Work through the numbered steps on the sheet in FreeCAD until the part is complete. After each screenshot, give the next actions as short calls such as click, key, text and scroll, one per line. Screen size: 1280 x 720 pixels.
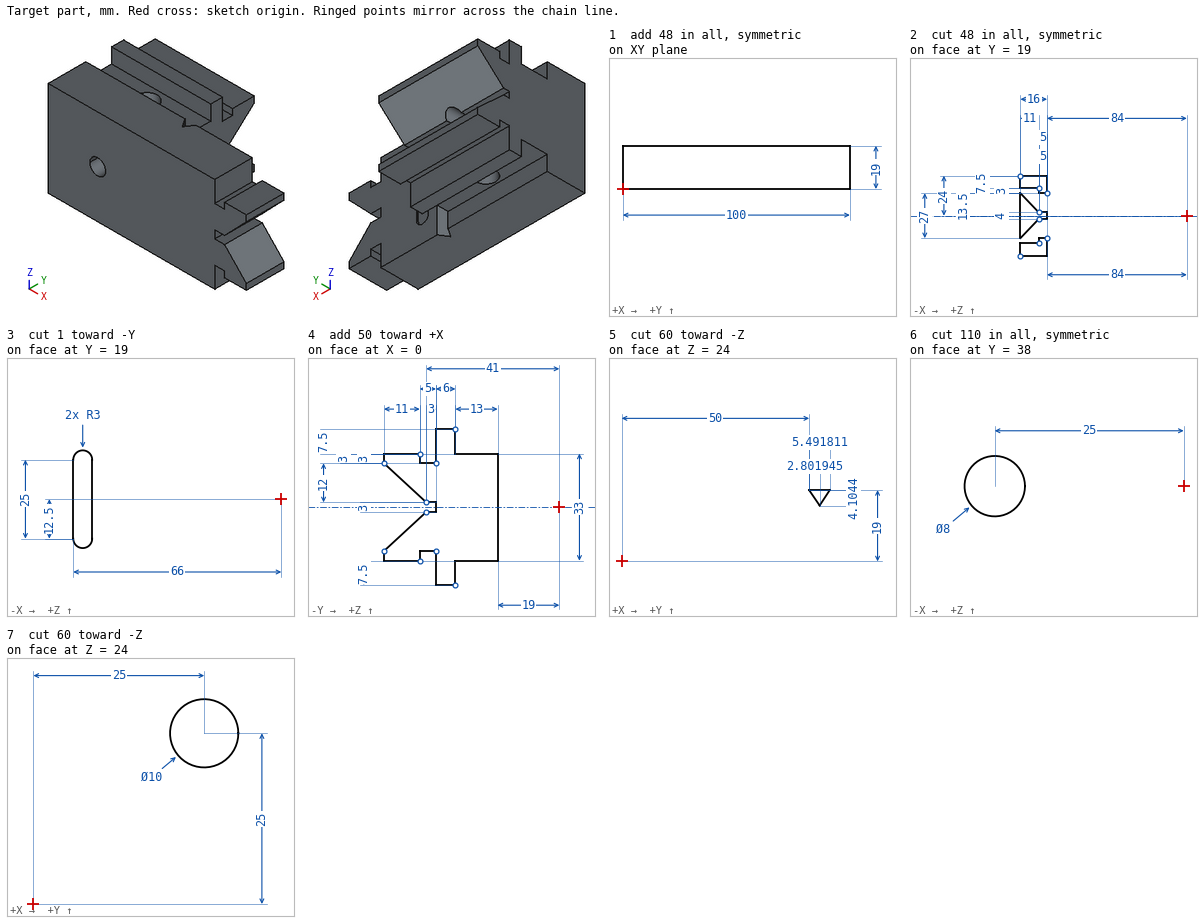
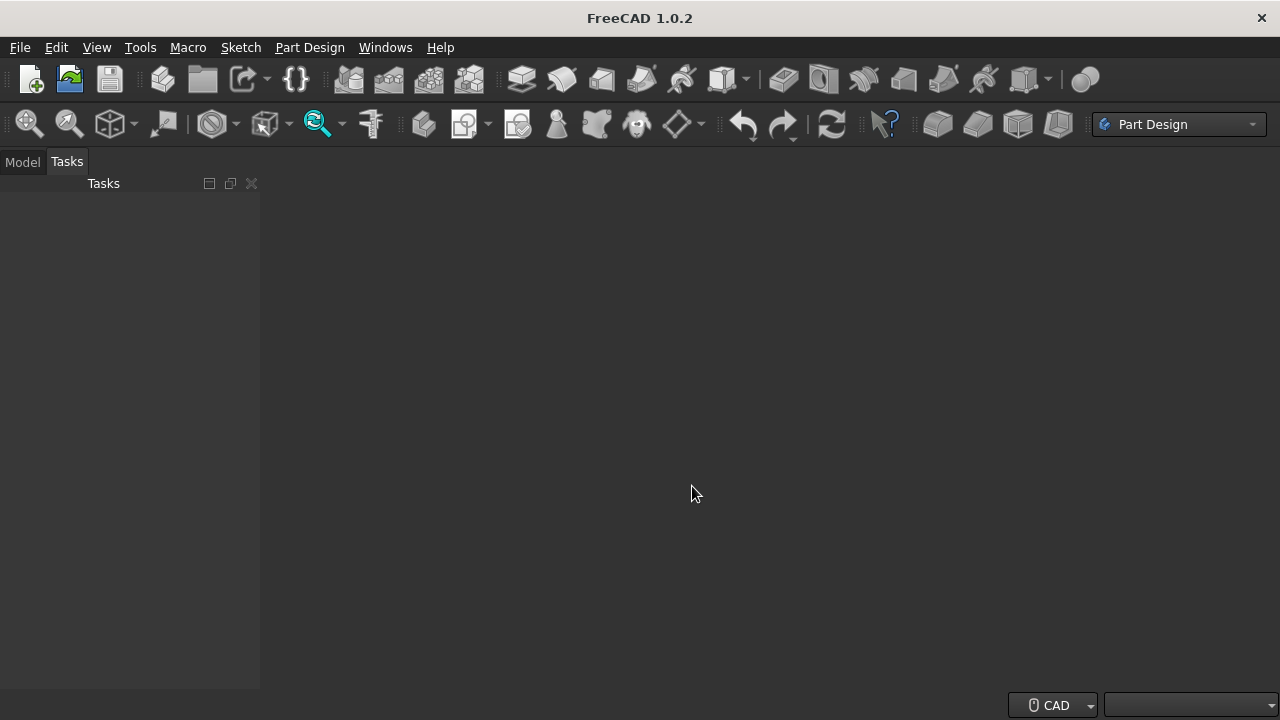
click(30, 80)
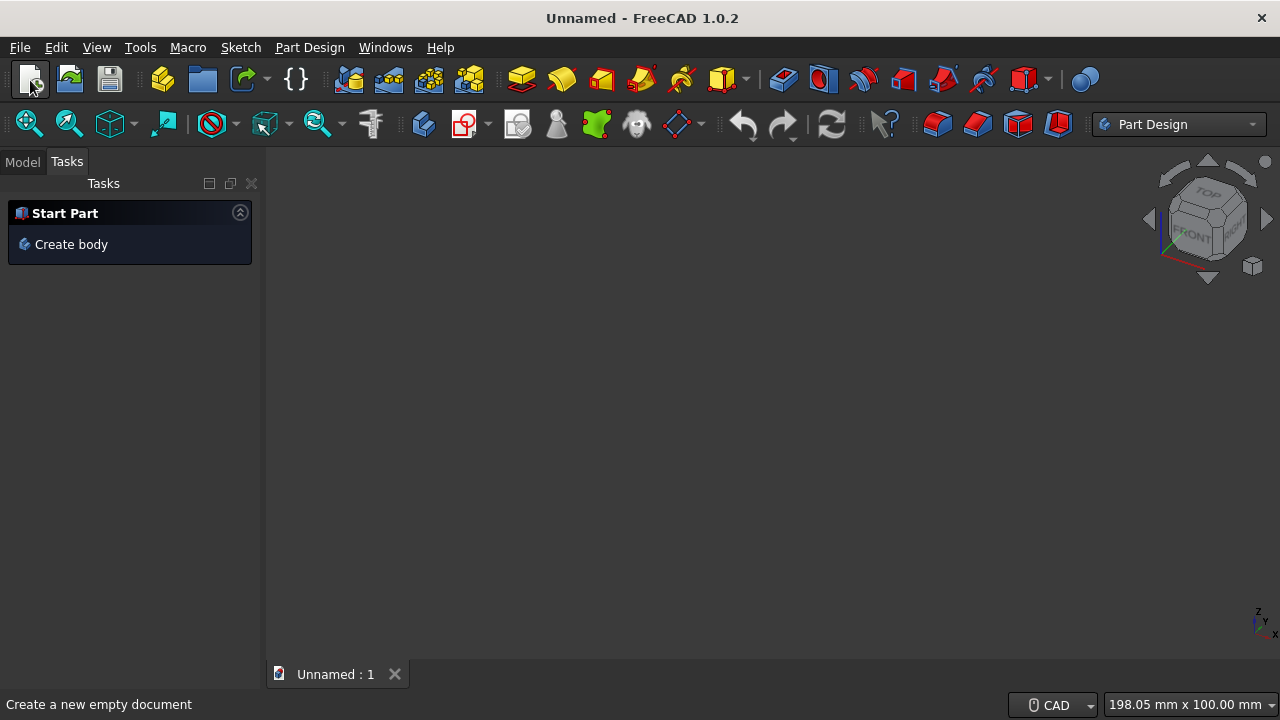
click(464, 124)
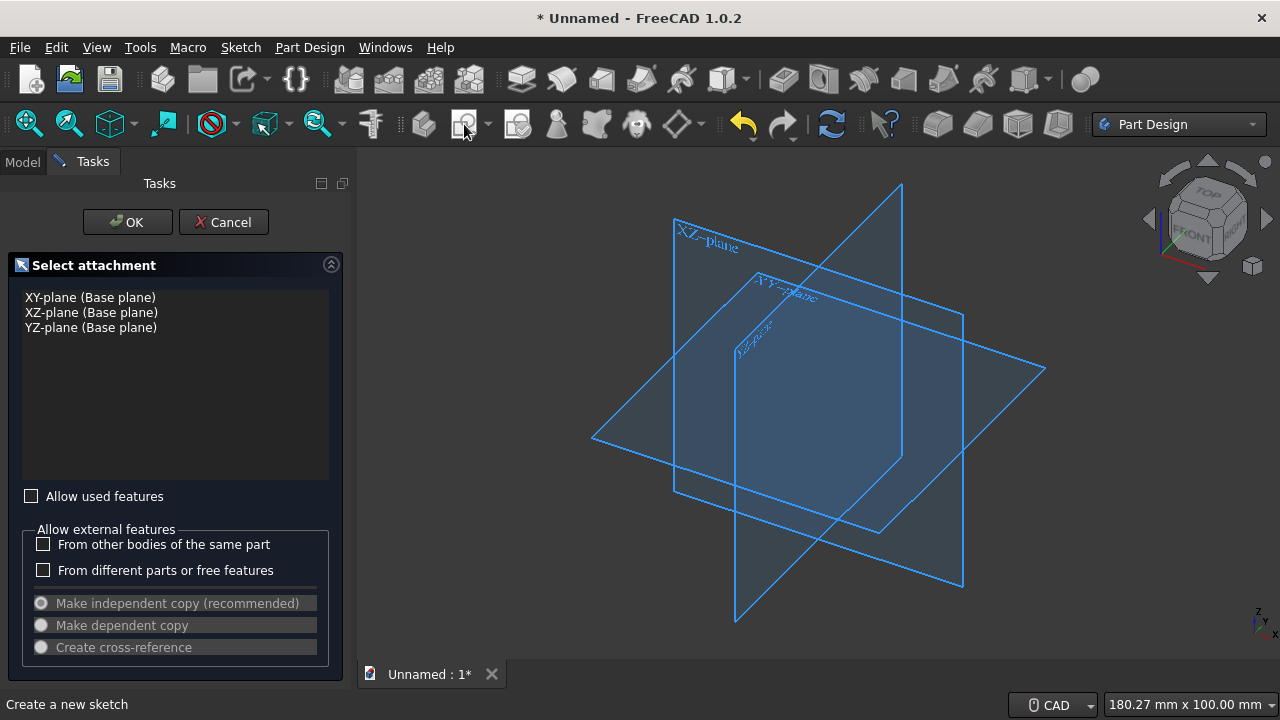
click(82, 298)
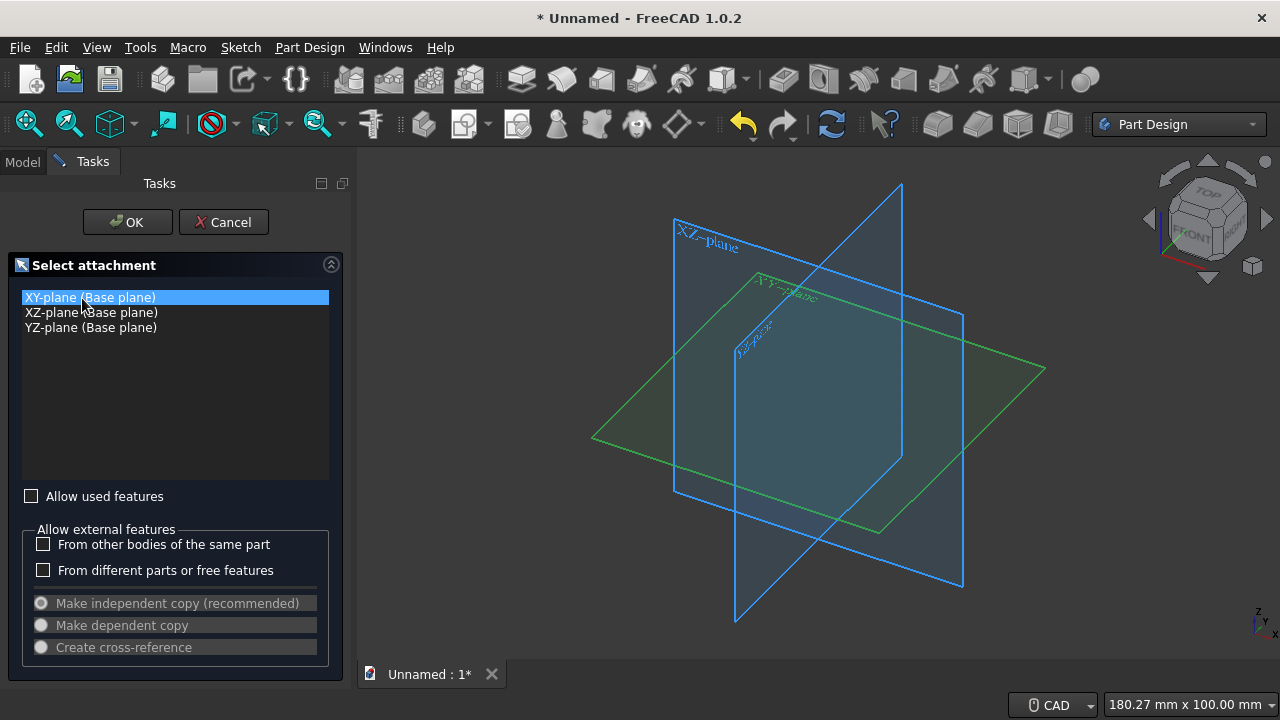
click(128, 222)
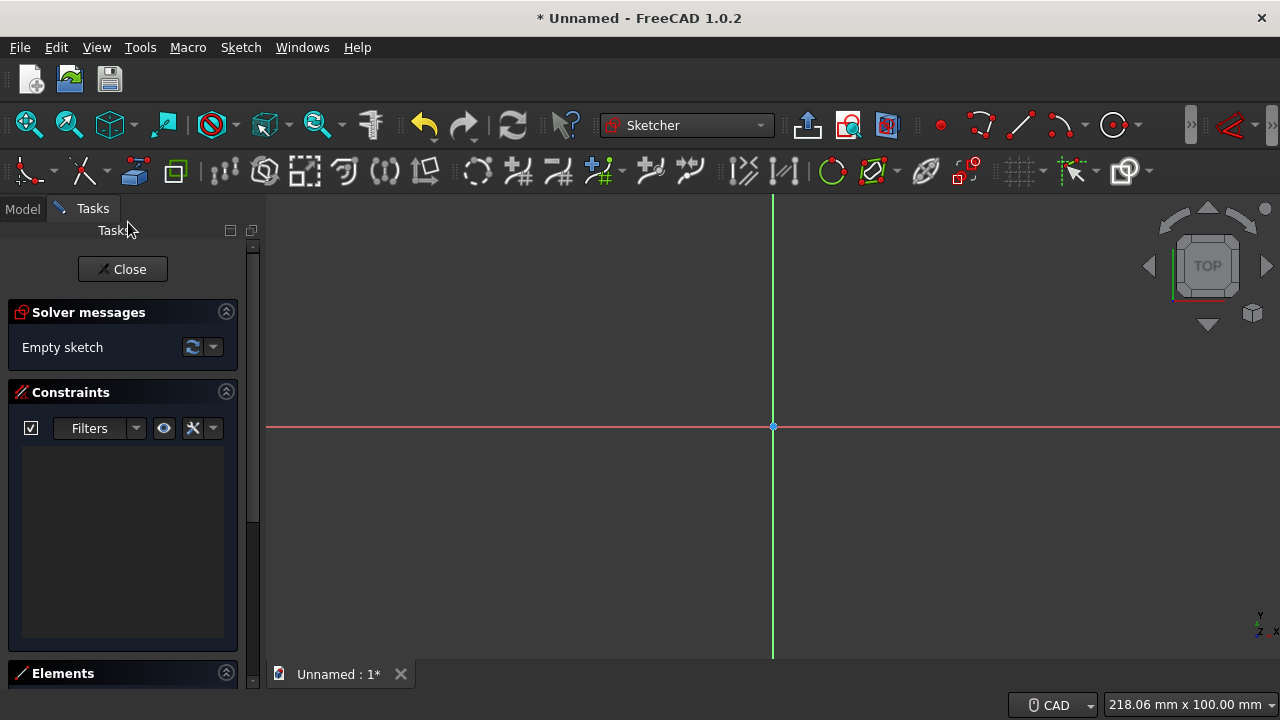
scroll(294, 626, down, 1)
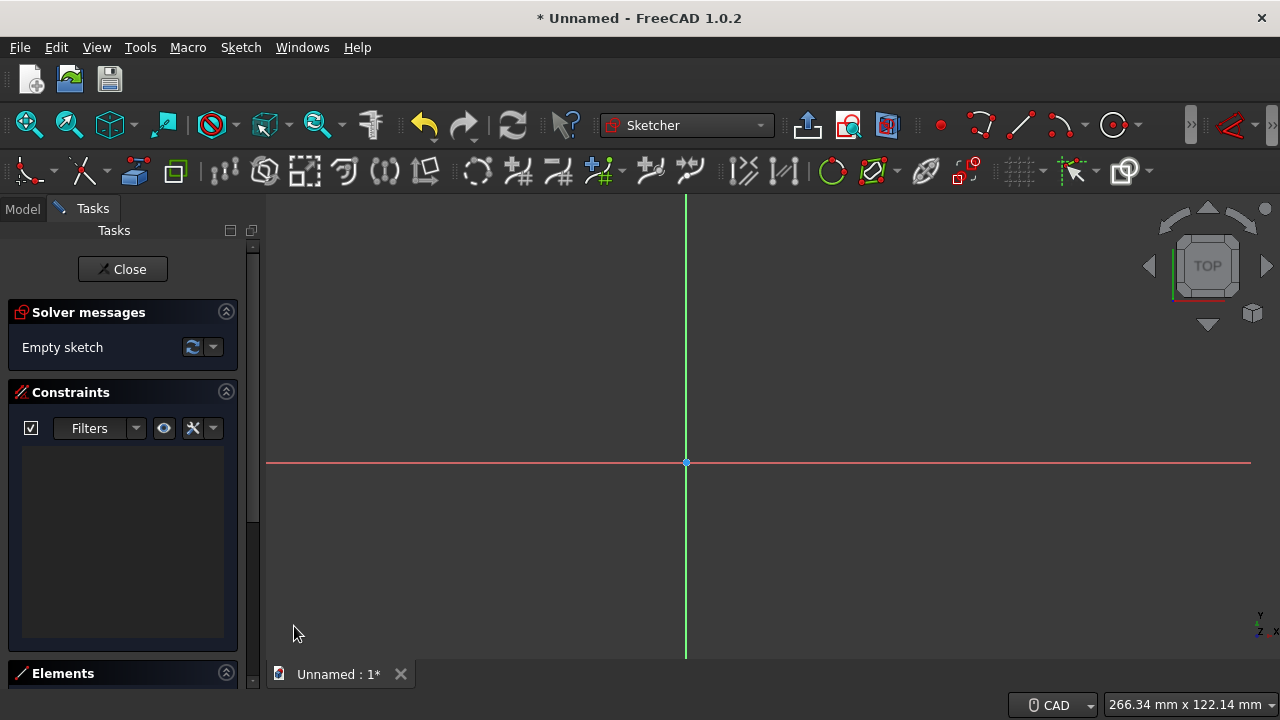
scroll(1115, 427, up, 2)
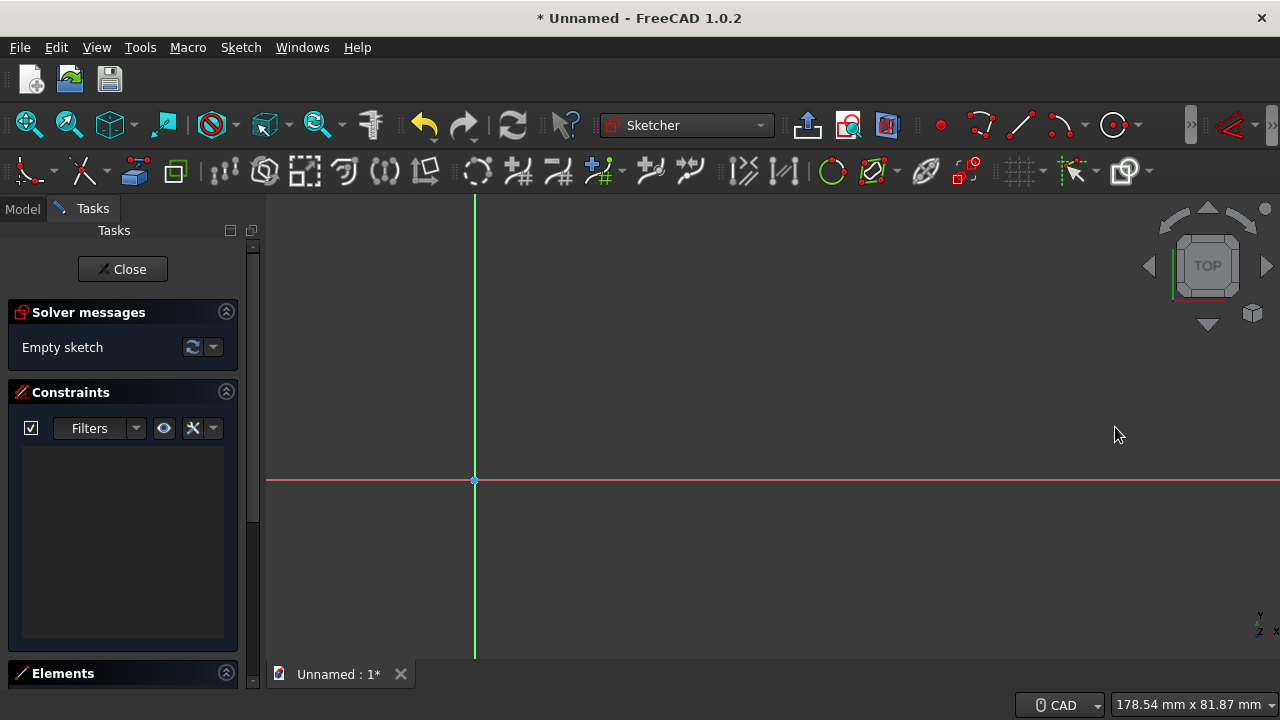
key(g)
key(r)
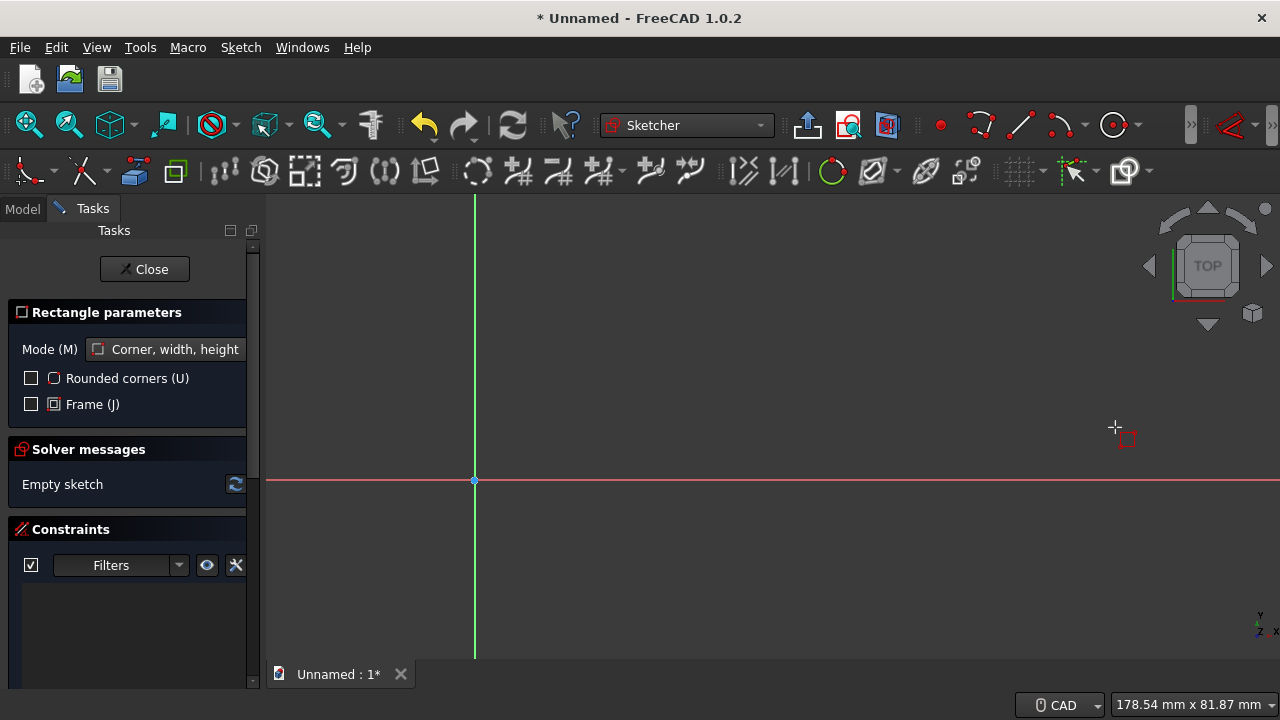
click(475, 480)
click(1043, 372)
key(Escape)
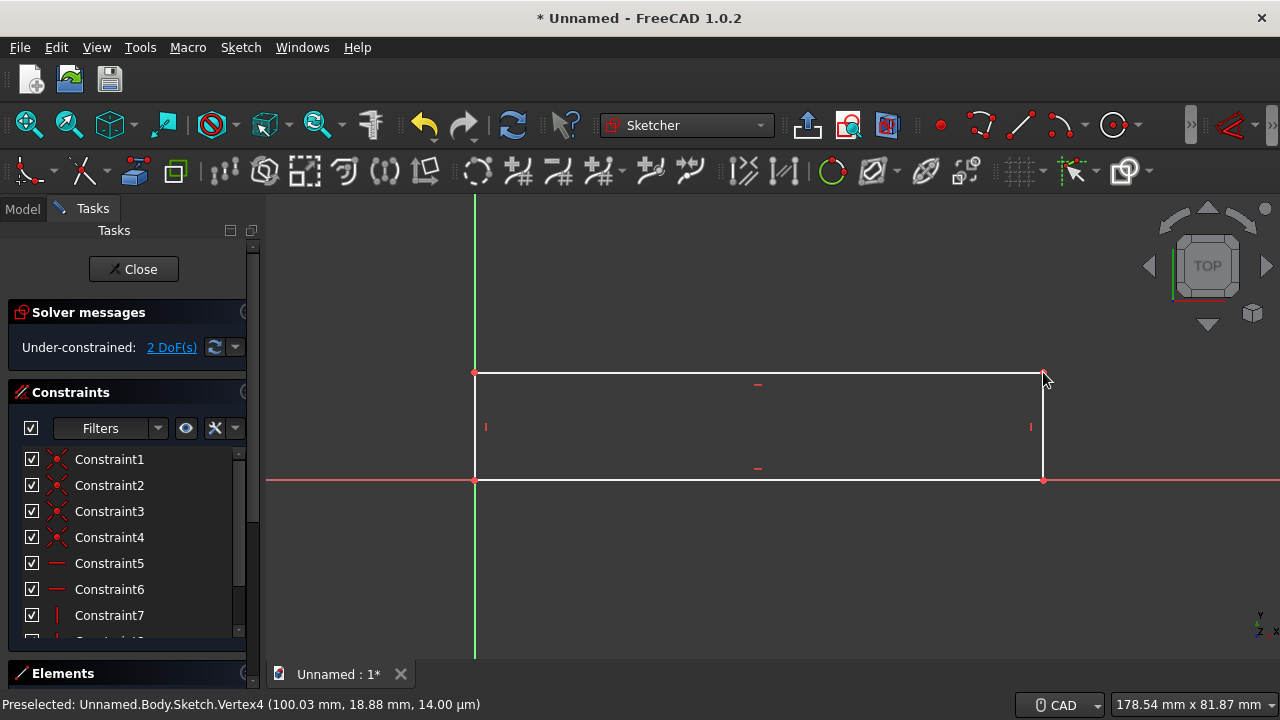
click(1230, 126)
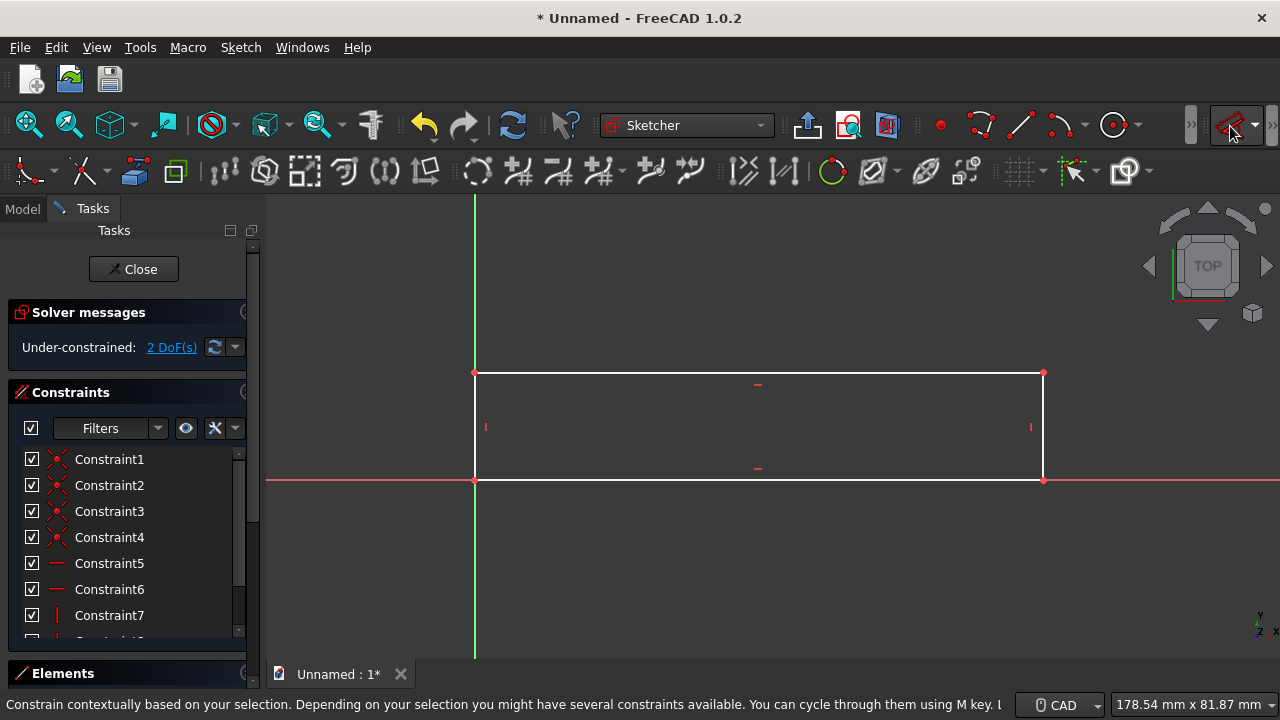
click(1043, 448)
click(1077, 427)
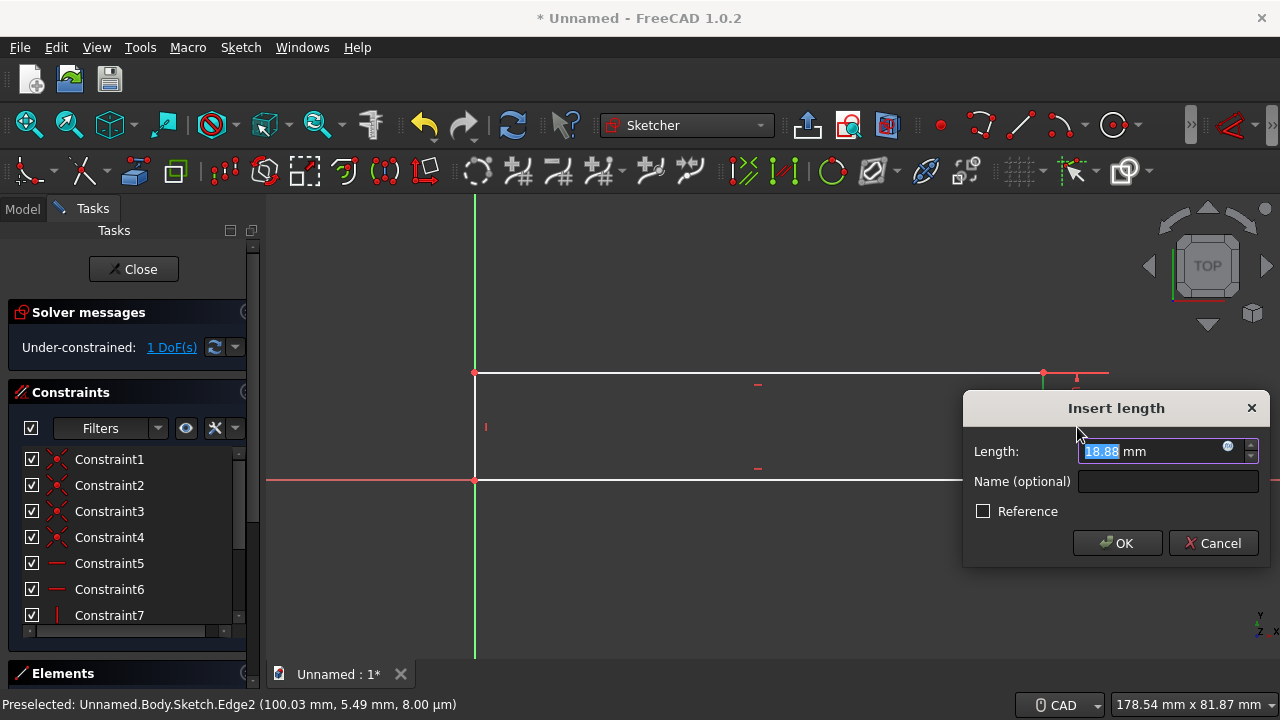
text(19)
key(Return)